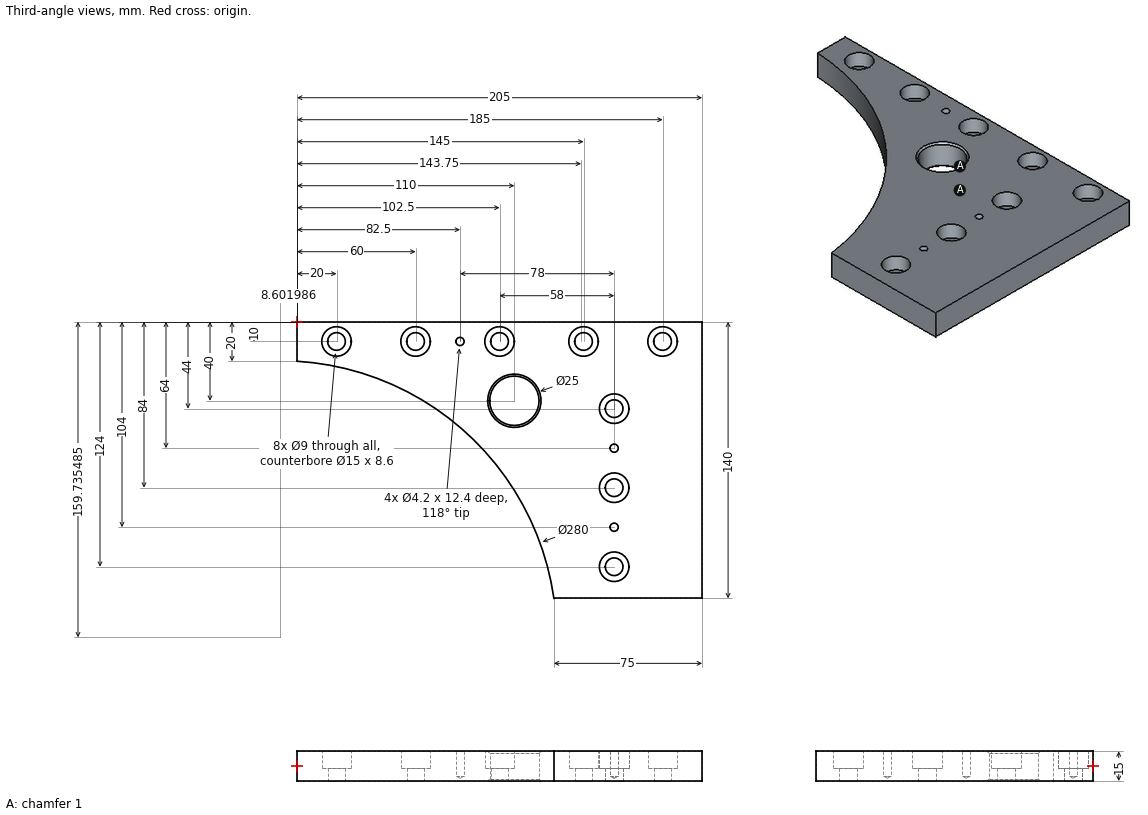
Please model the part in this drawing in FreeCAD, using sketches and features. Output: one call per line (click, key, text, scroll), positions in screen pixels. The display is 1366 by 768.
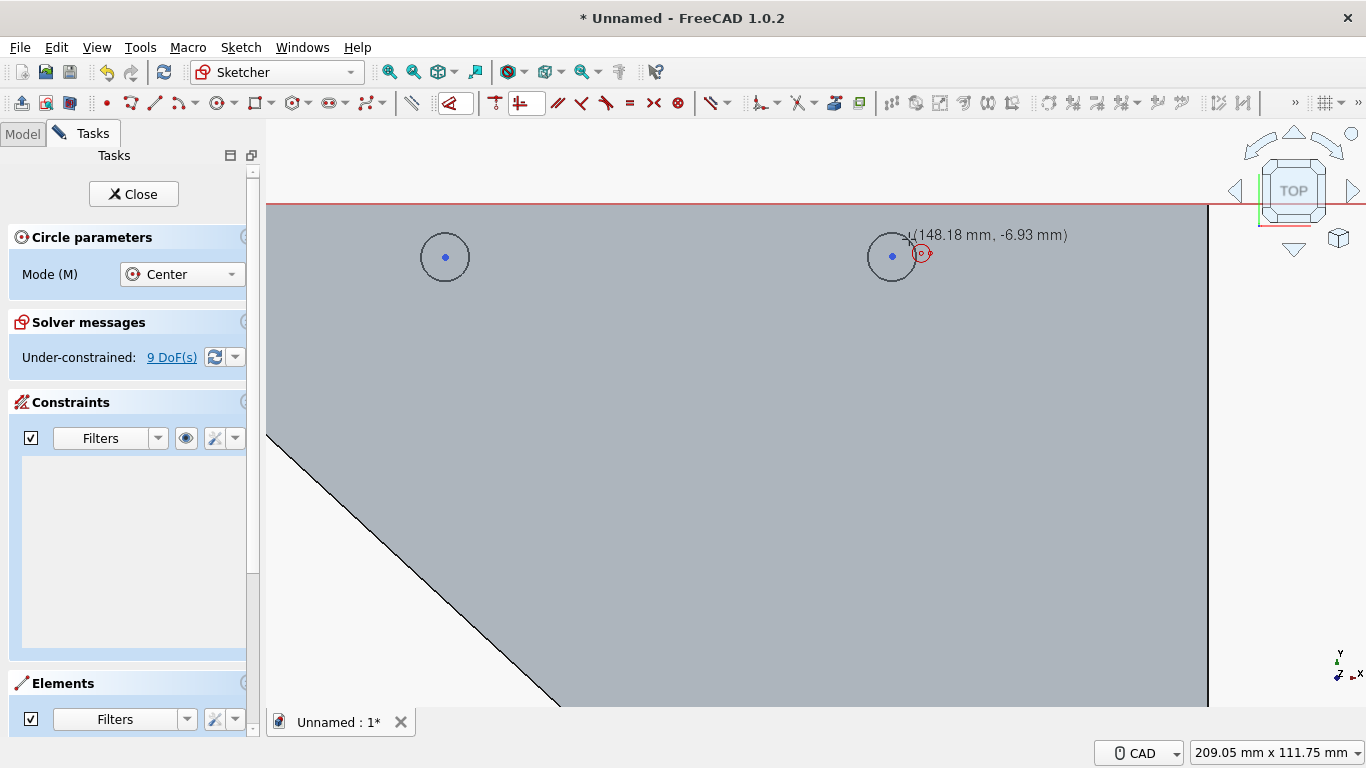
click(669, 256)
click(685, 239)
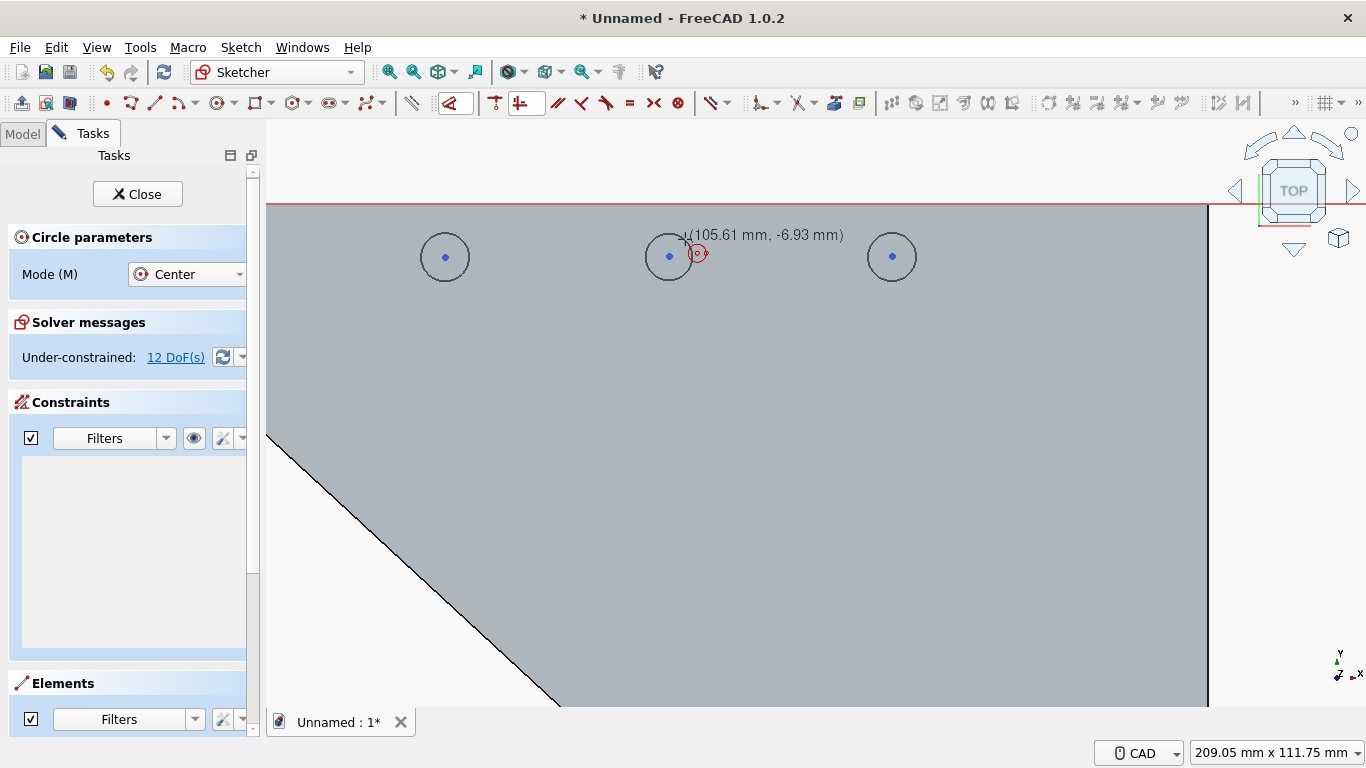
click(1103, 256)
click(1120, 239)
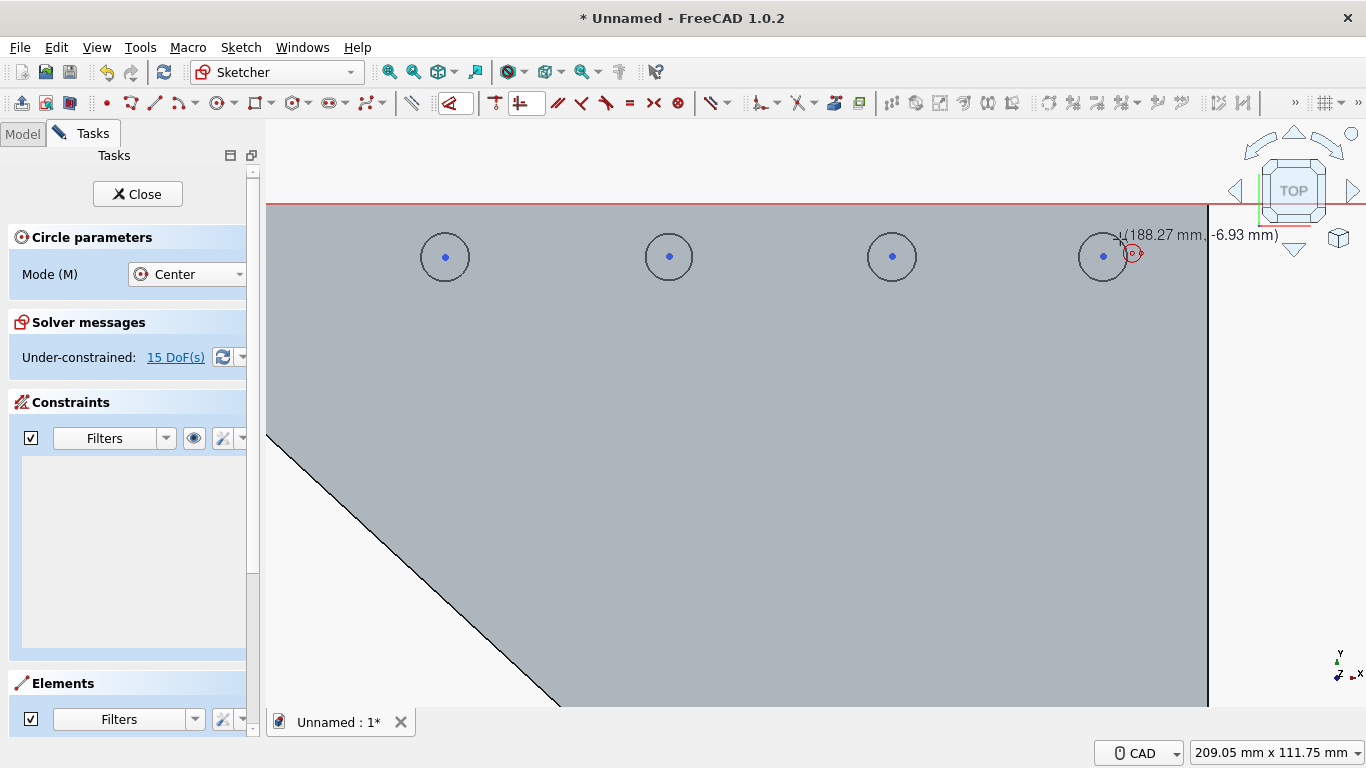
click(974, 435)
click(991, 418)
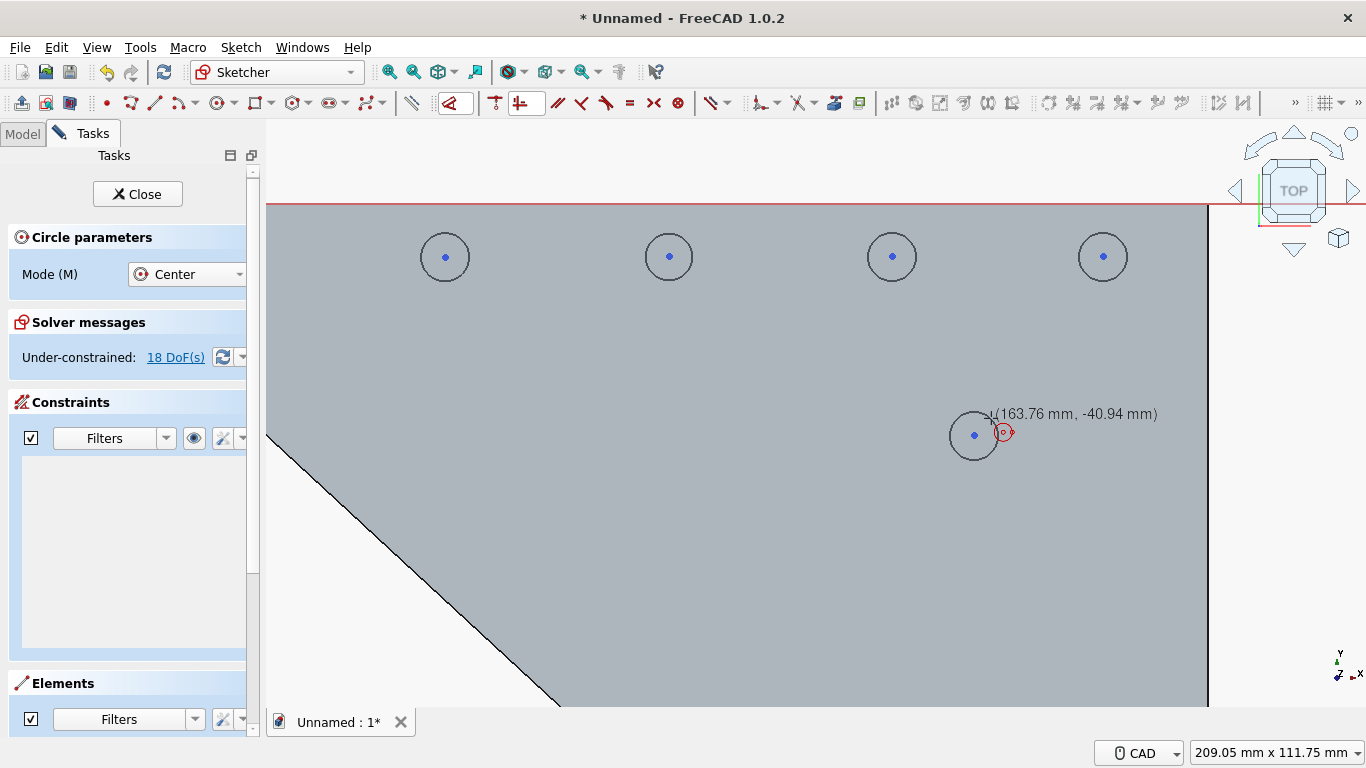
click(974, 646)
click(991, 629)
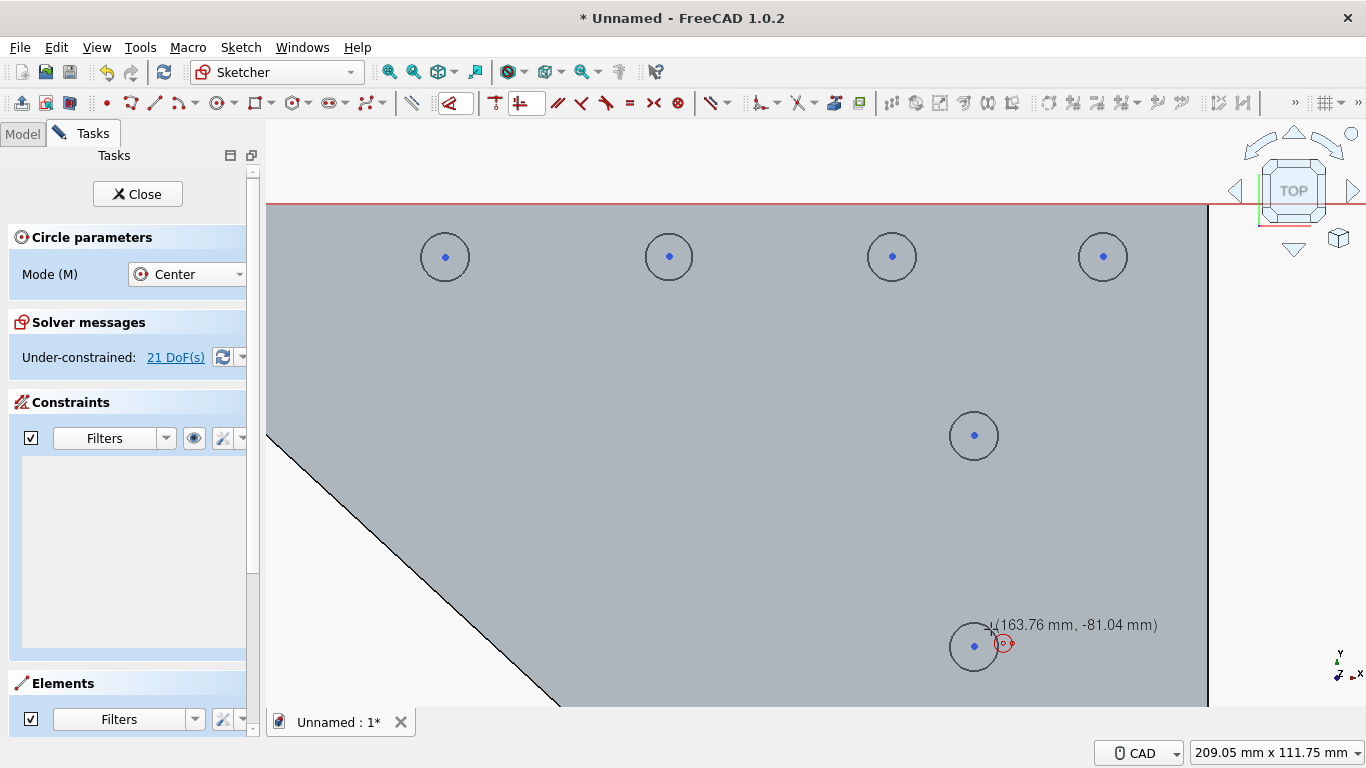
scroll(893, 257, down, 3)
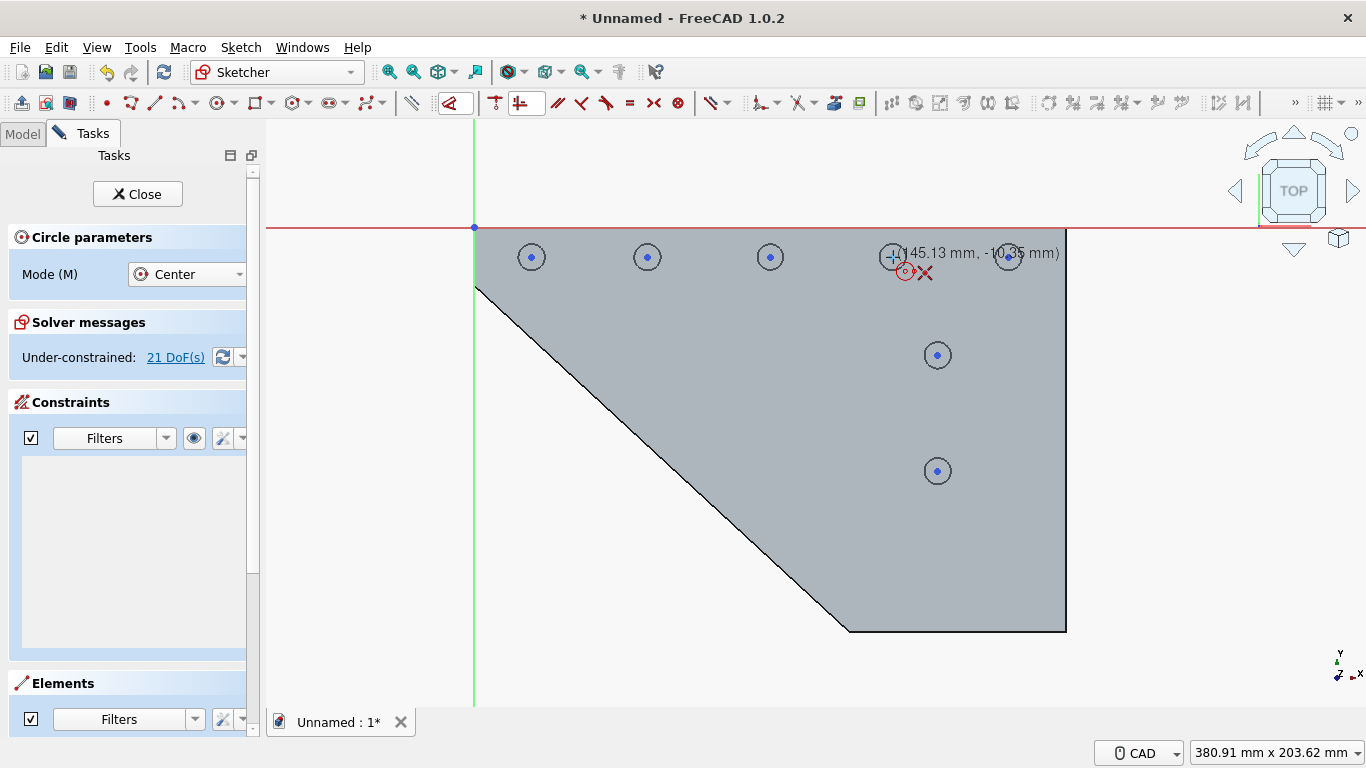
scroll(938, 586, up, 3)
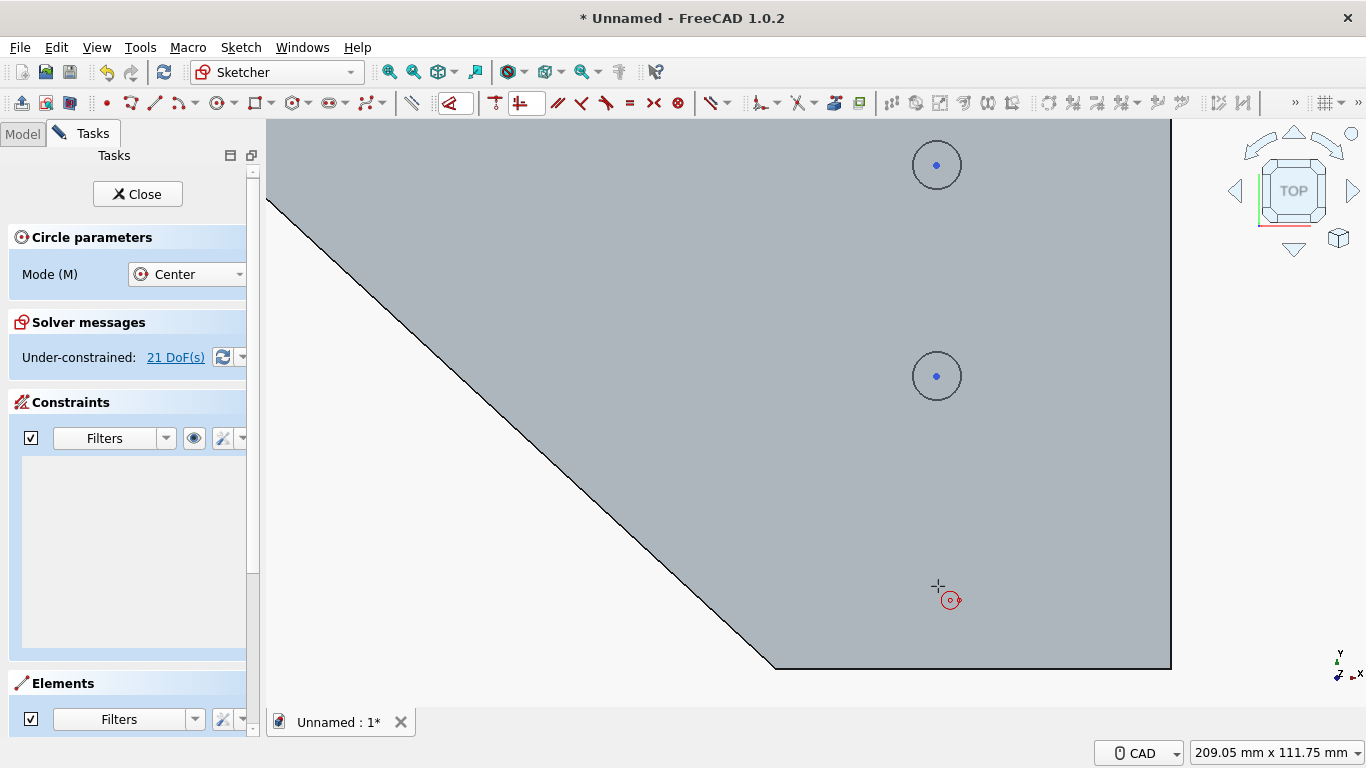
click(937, 585)
click(954, 568)
key(Escape)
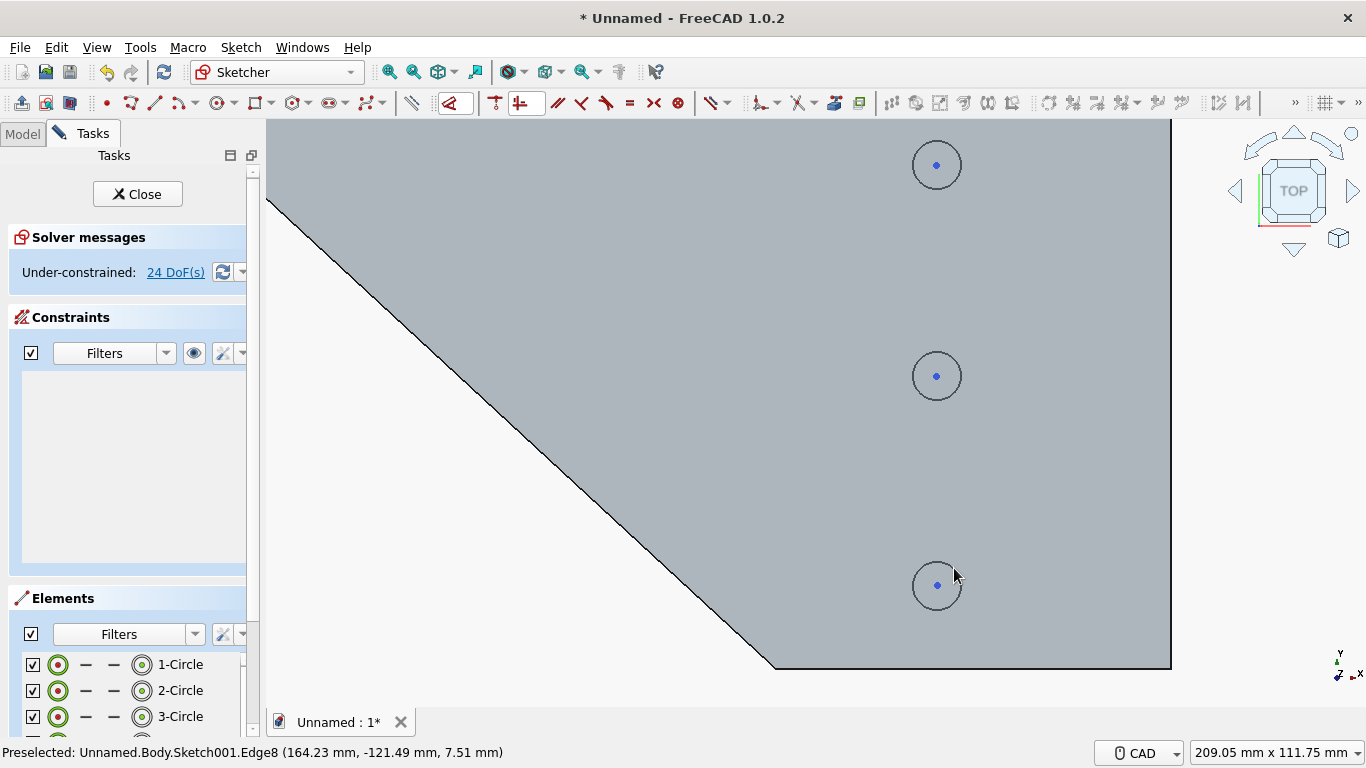
scroll(938, 586, down, 3)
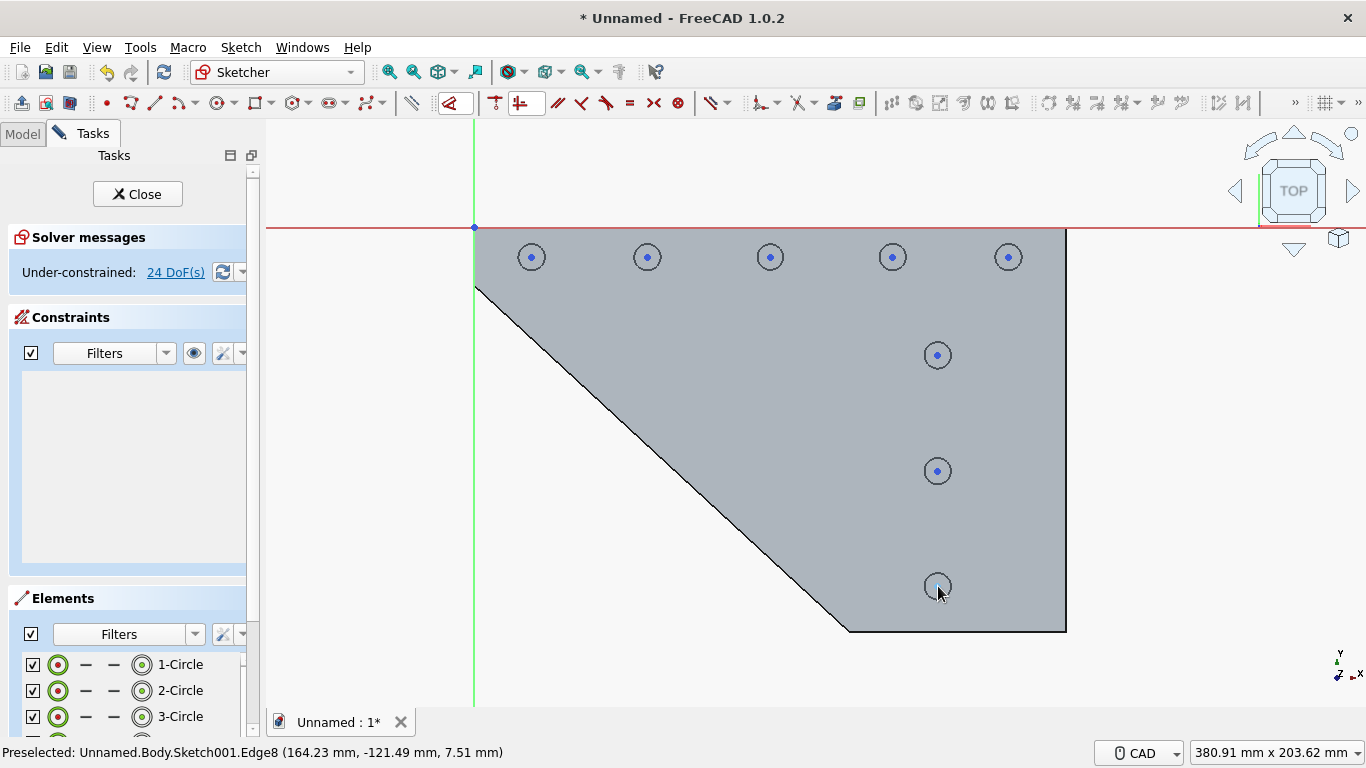
click(541, 248)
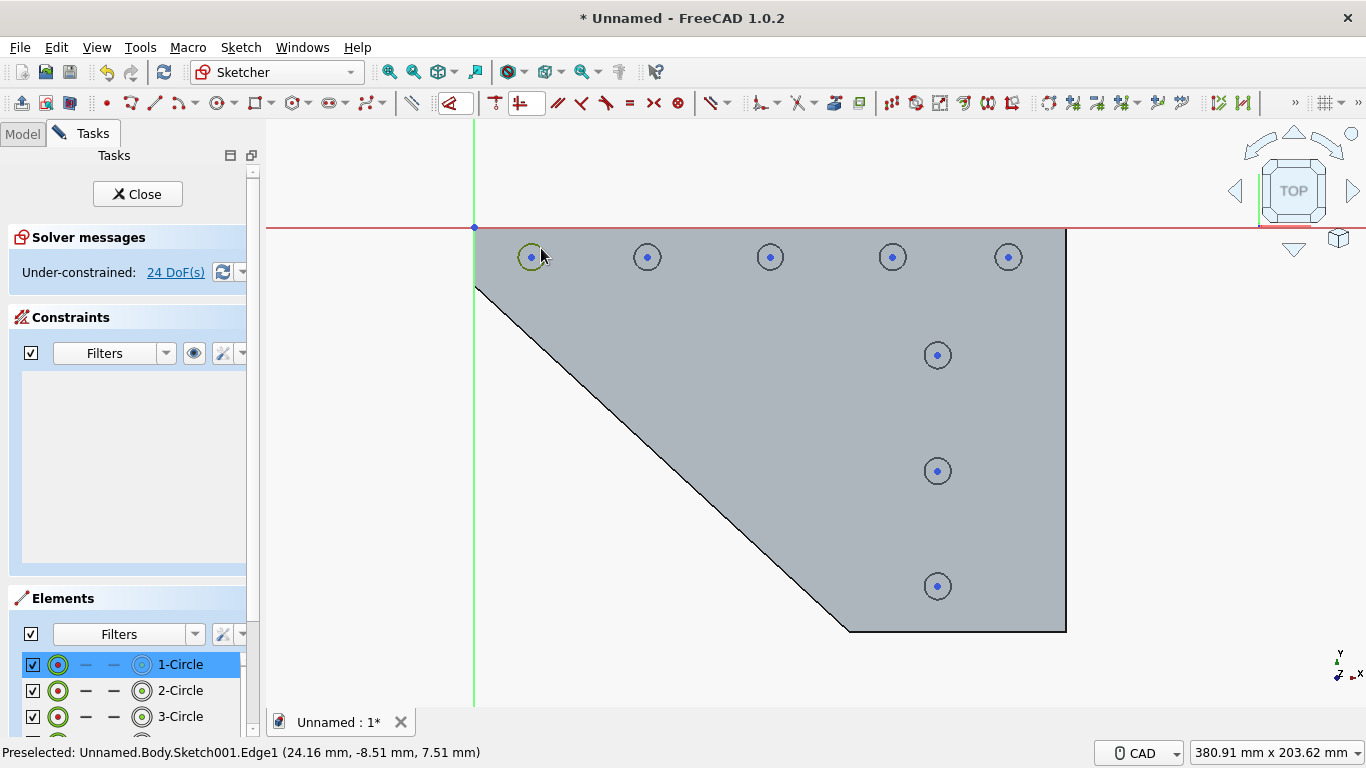
click(657, 248)